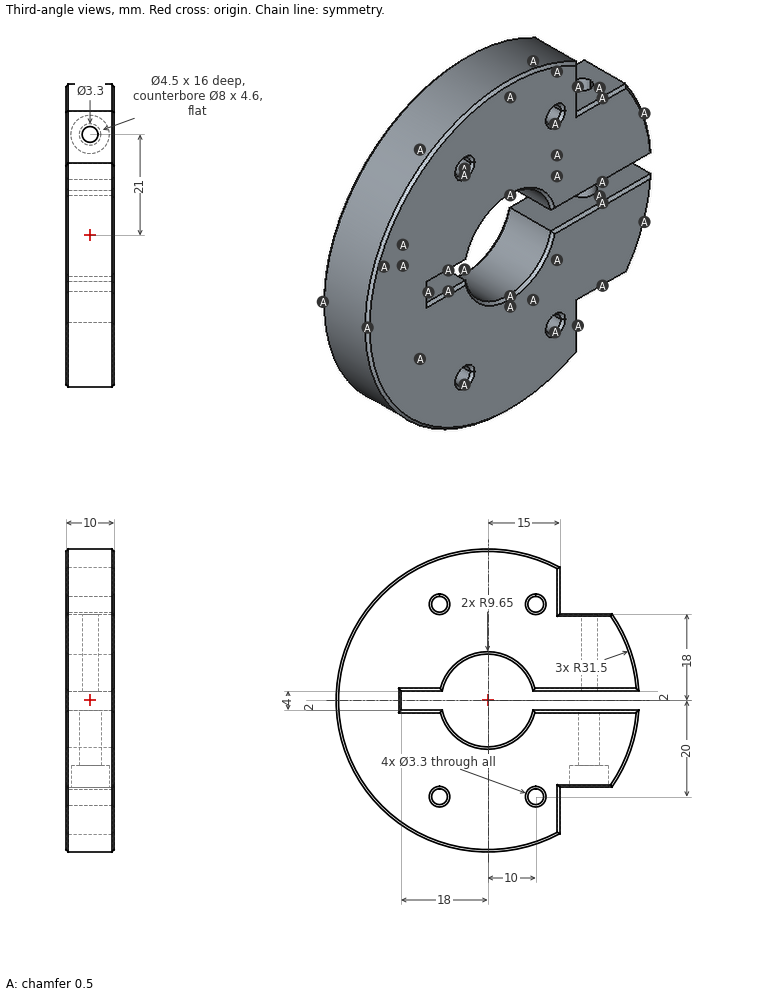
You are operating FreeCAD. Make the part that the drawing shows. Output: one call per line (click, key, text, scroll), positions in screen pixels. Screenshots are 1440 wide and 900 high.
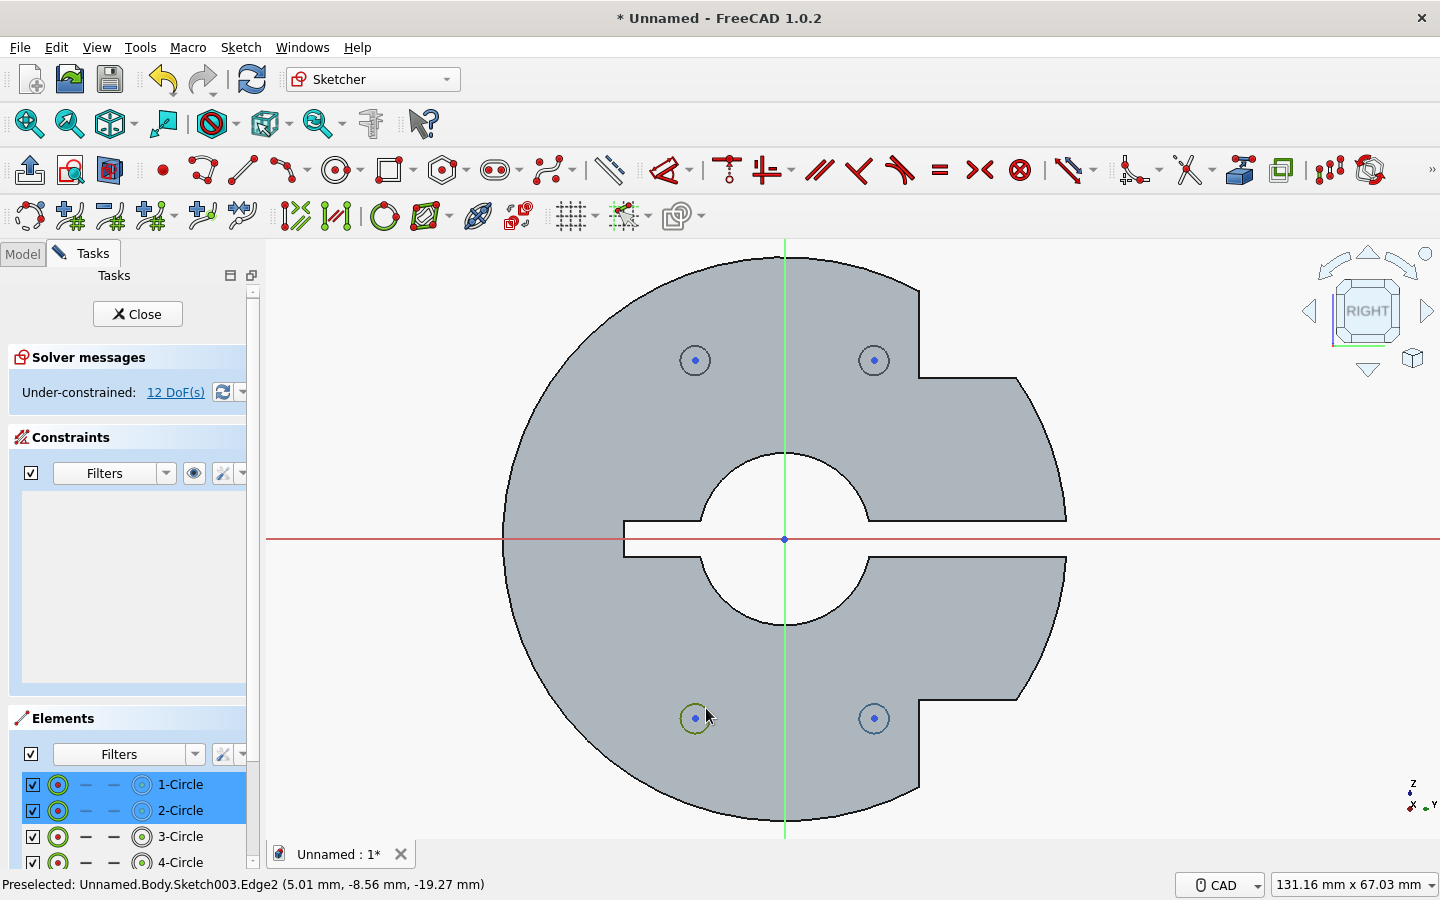
click(706, 350)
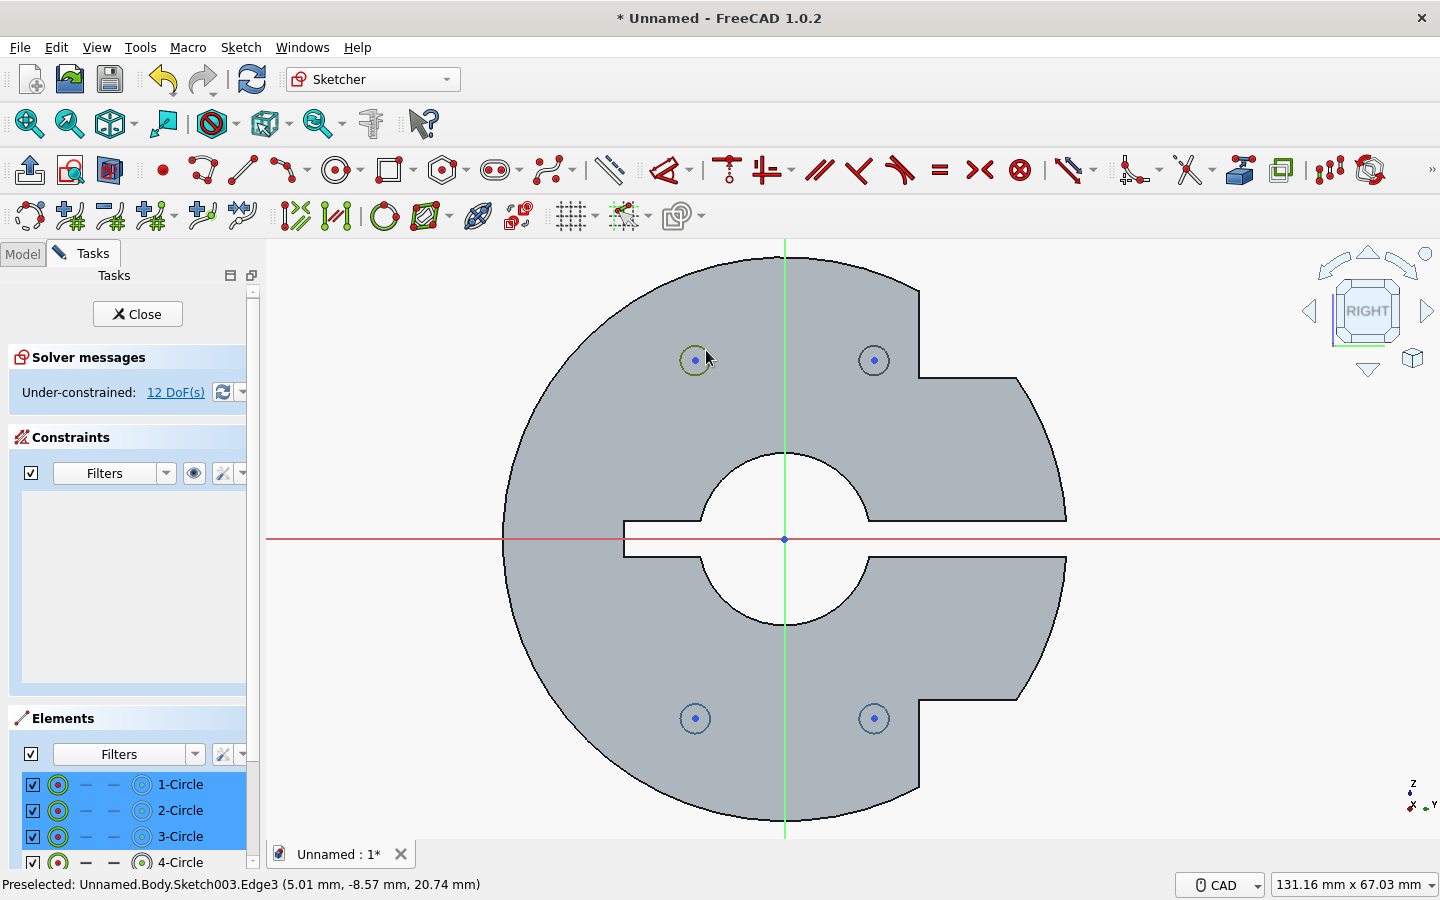
click(884, 350)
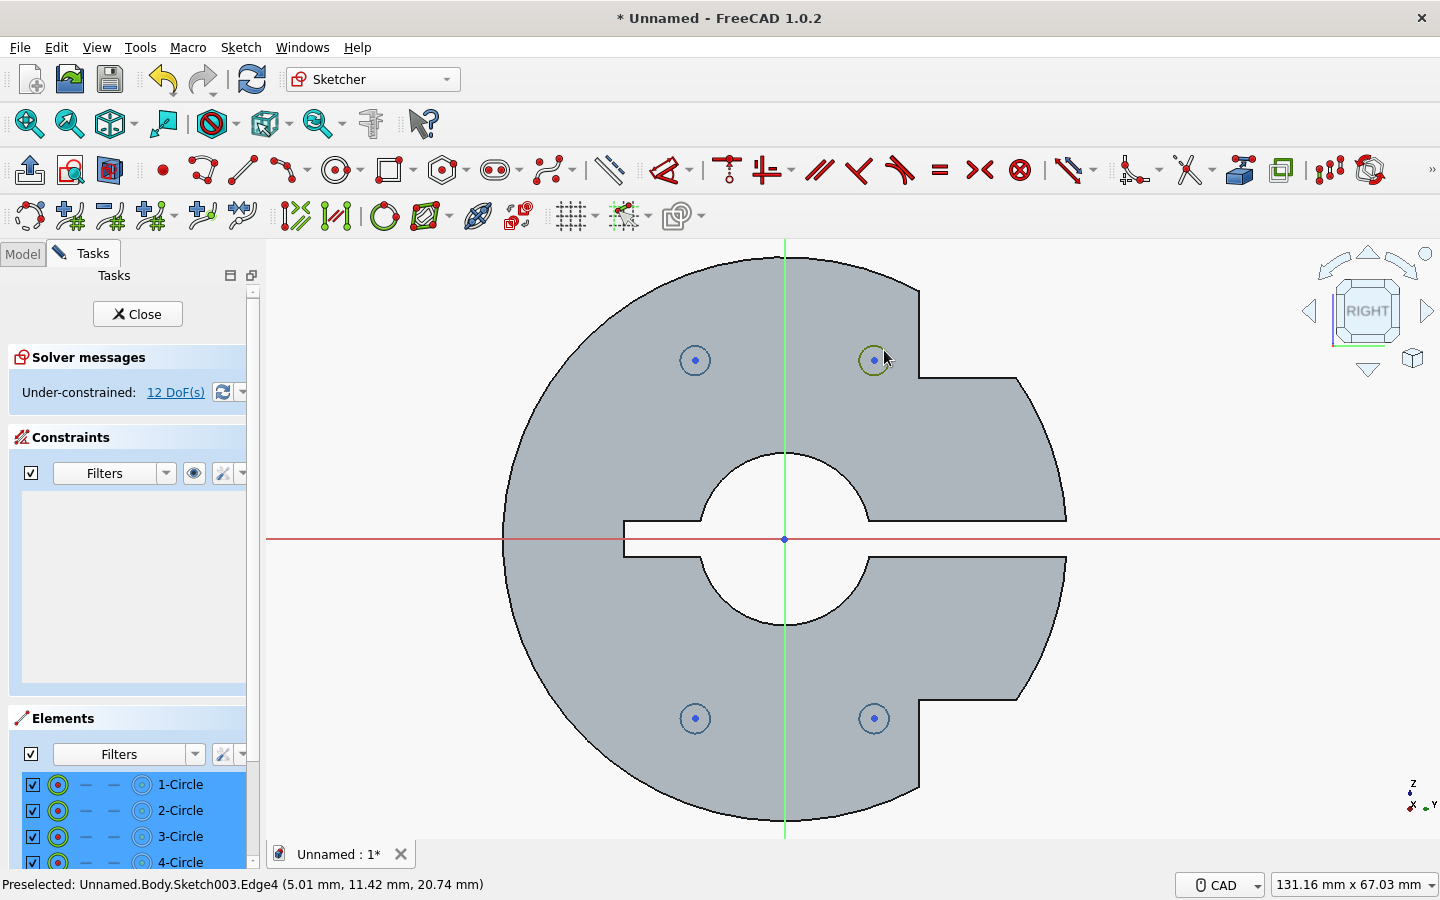
key(e)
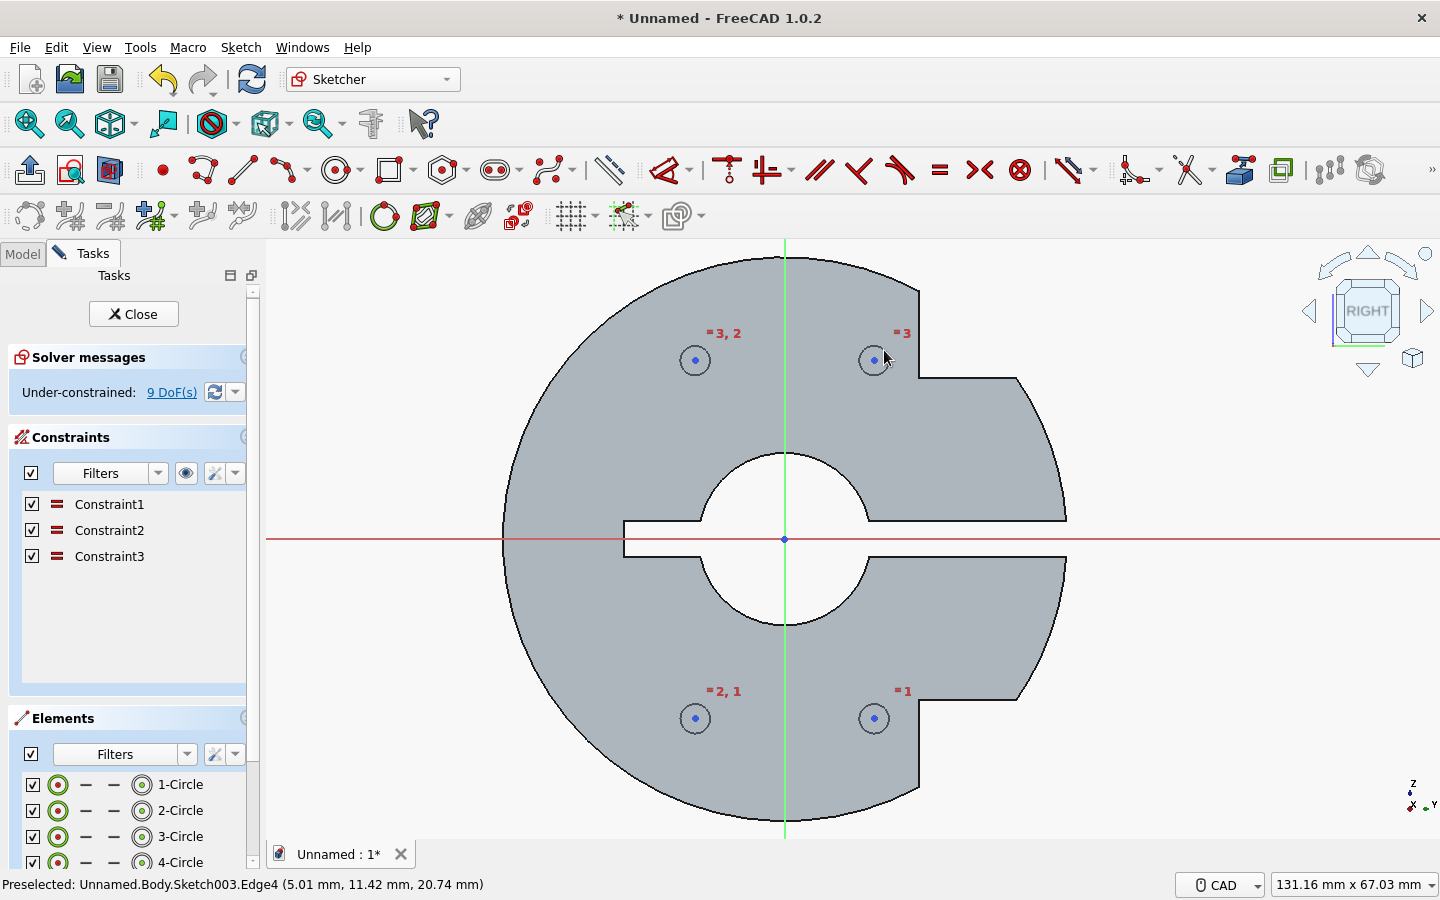
click(874, 719)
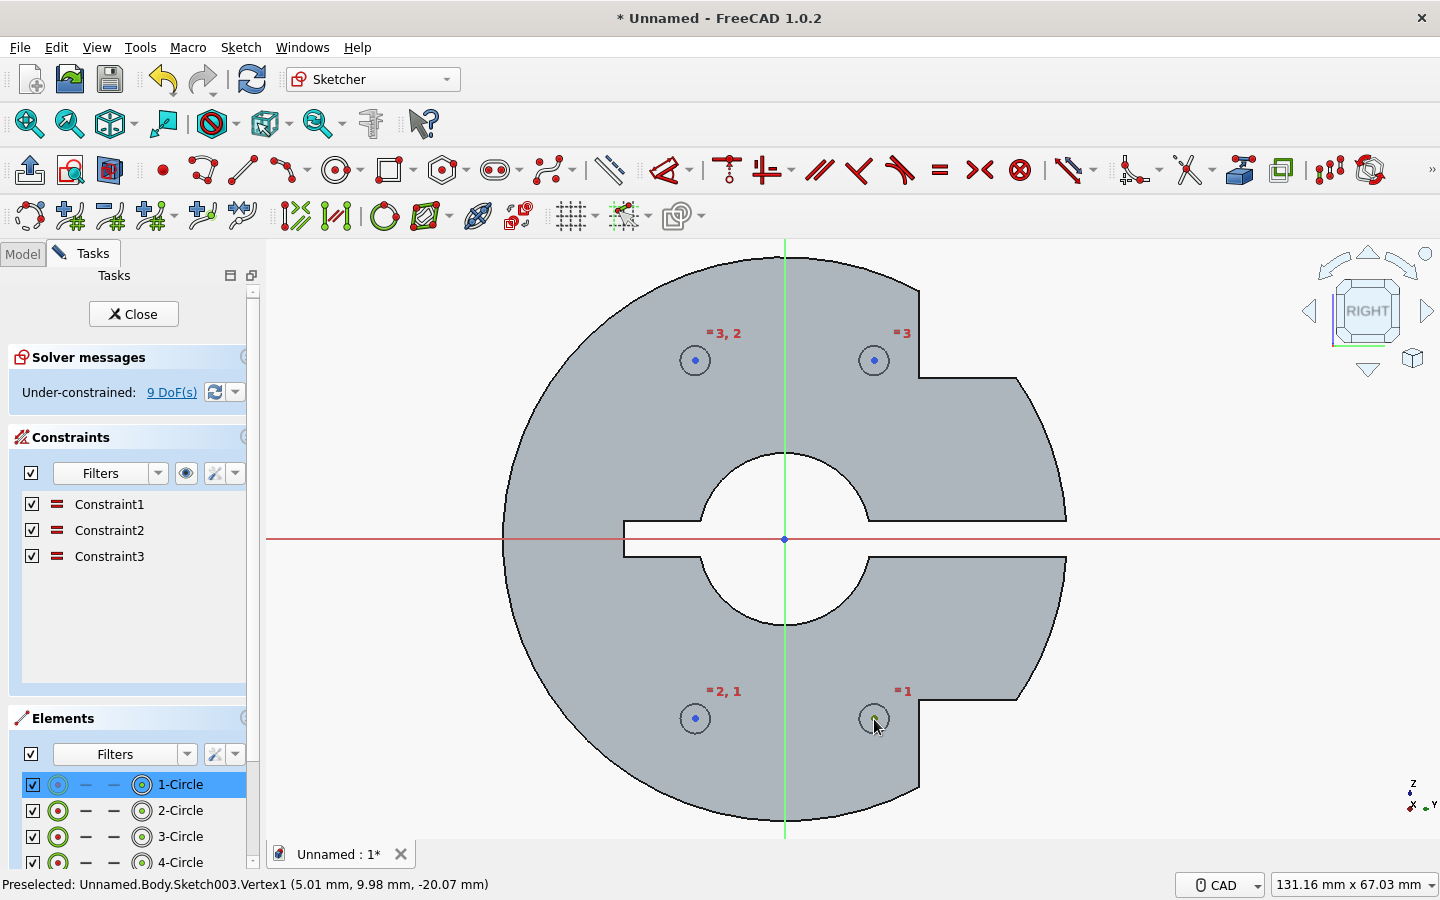
click(695, 719)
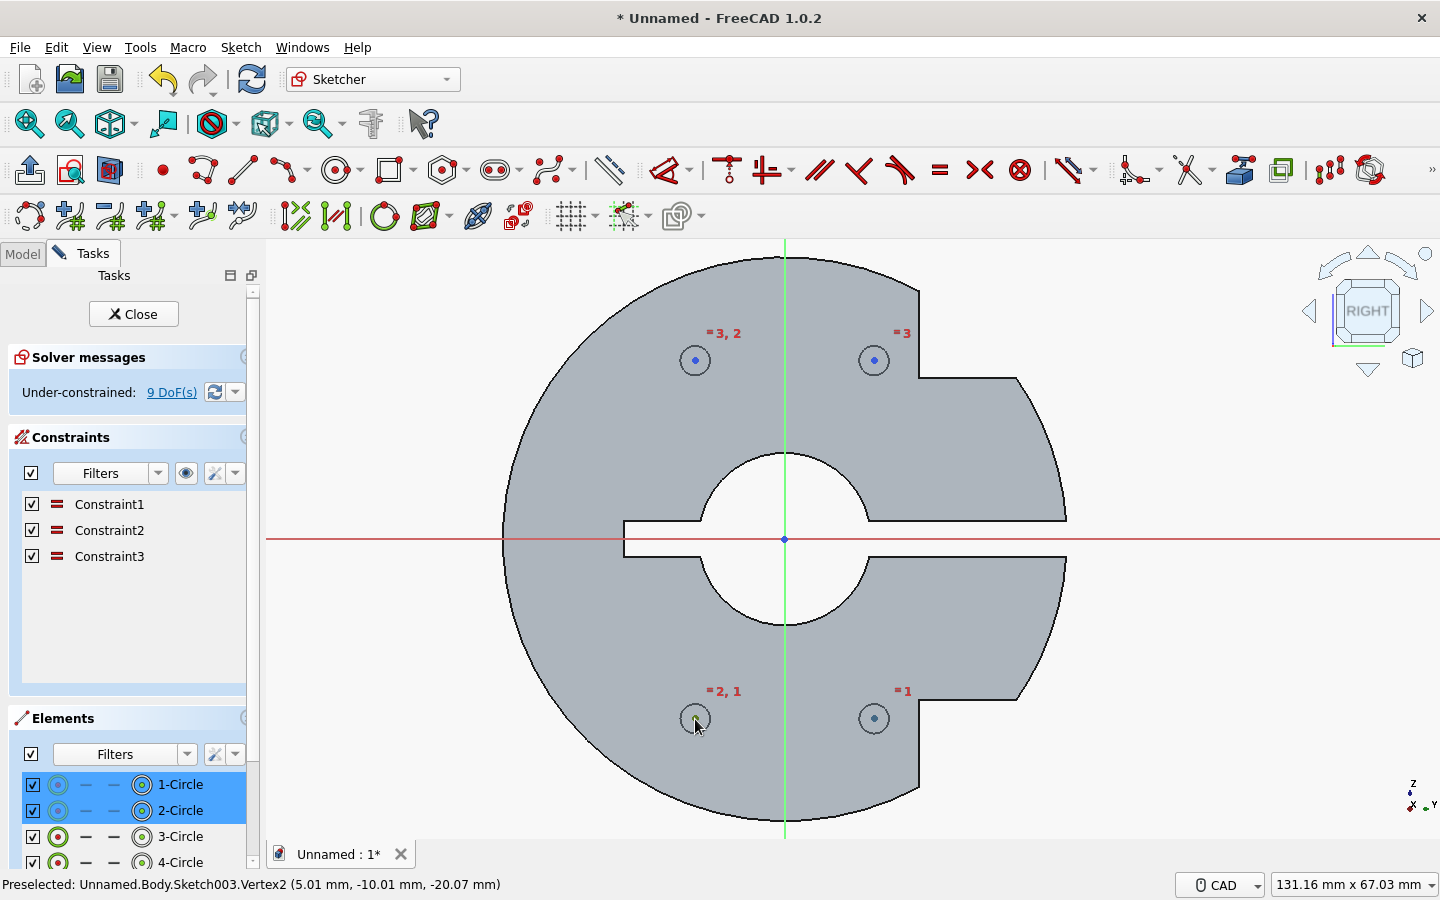
click(785, 772)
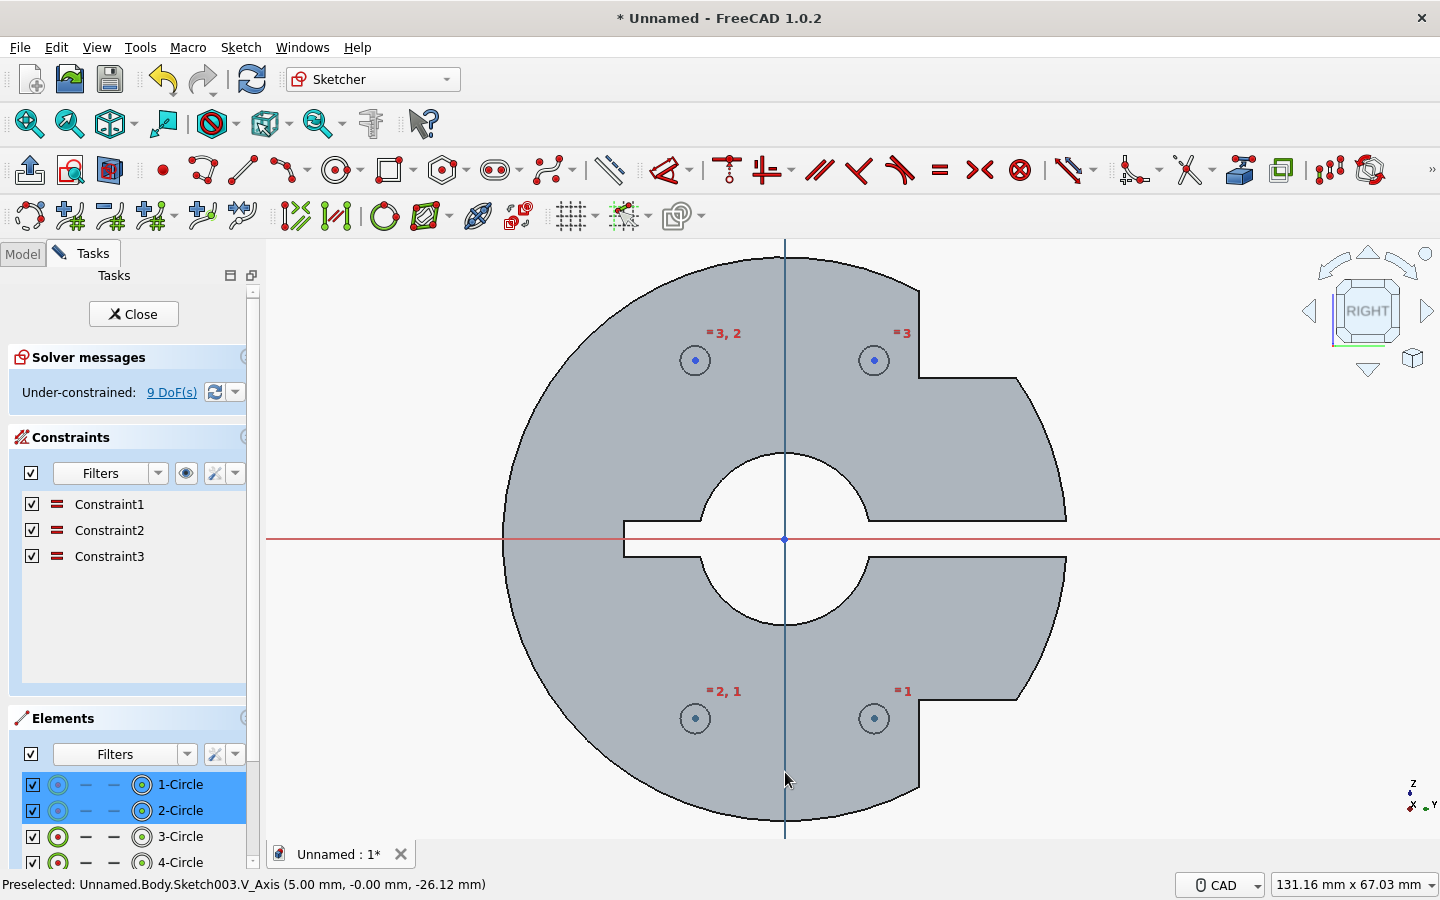
key(s)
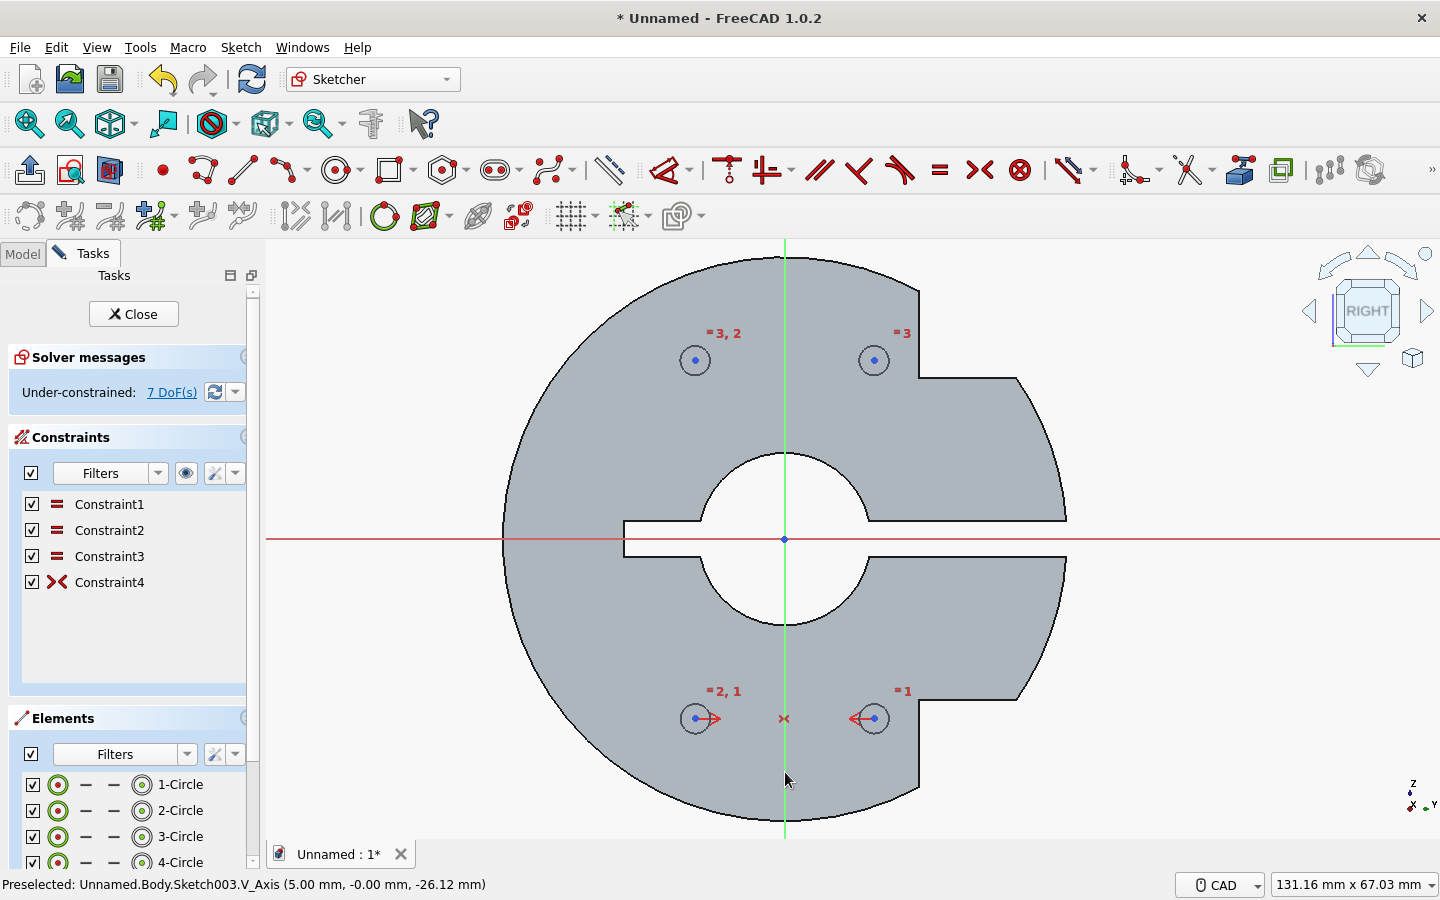
click(695, 719)